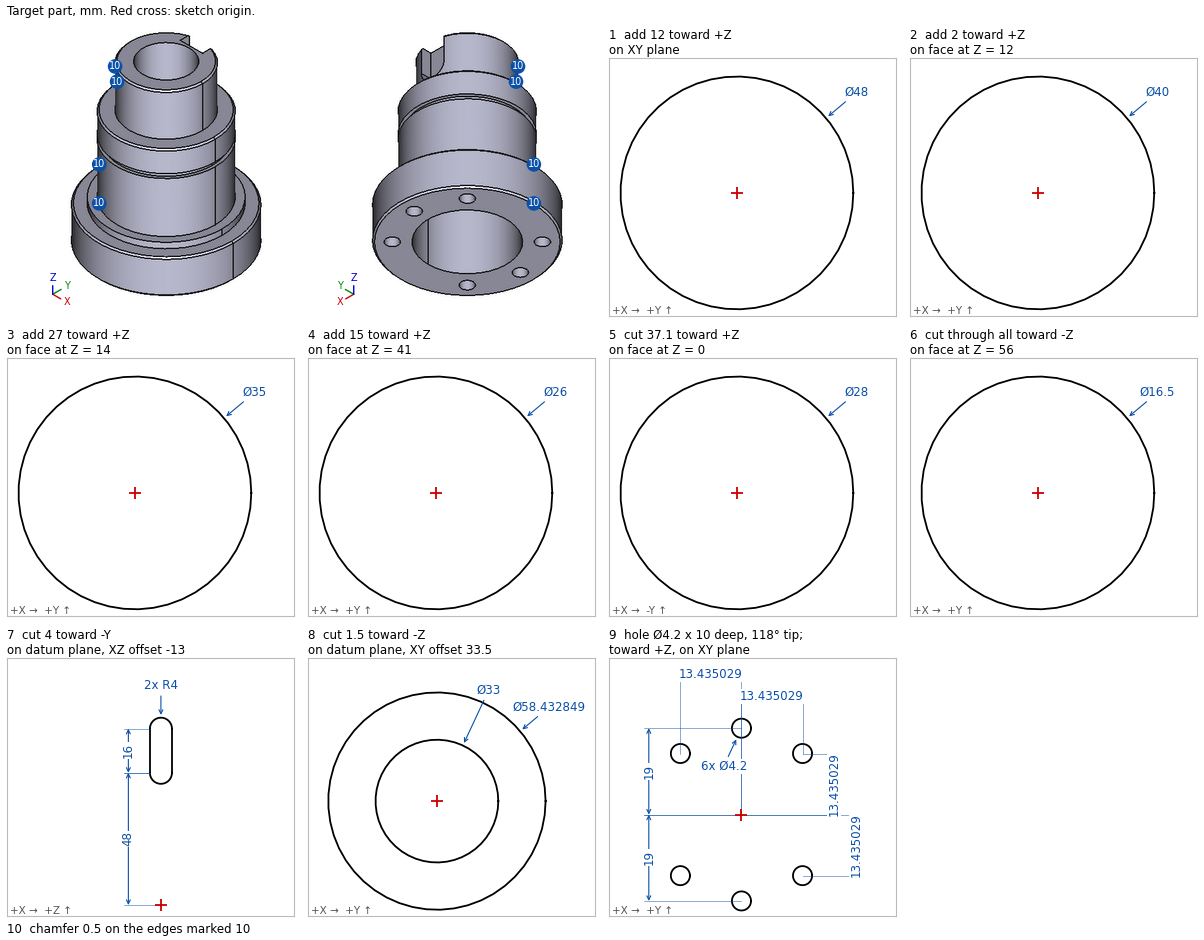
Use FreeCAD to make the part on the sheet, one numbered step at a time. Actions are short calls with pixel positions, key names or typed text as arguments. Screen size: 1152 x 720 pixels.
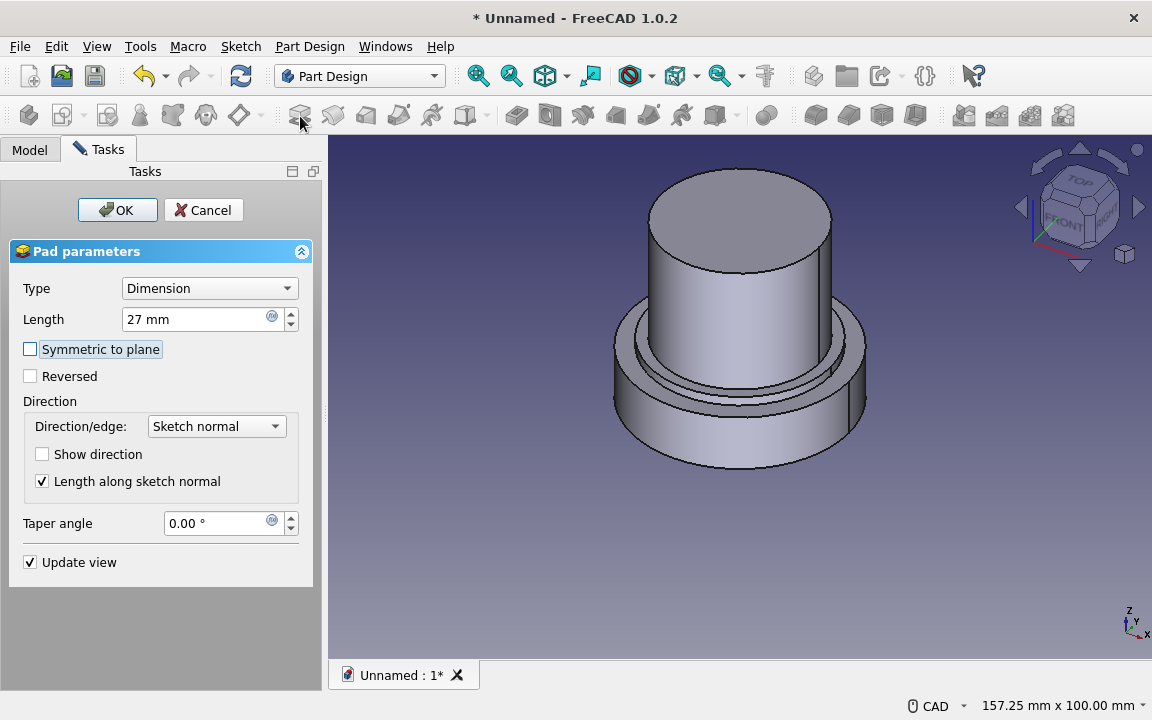
click(118, 210)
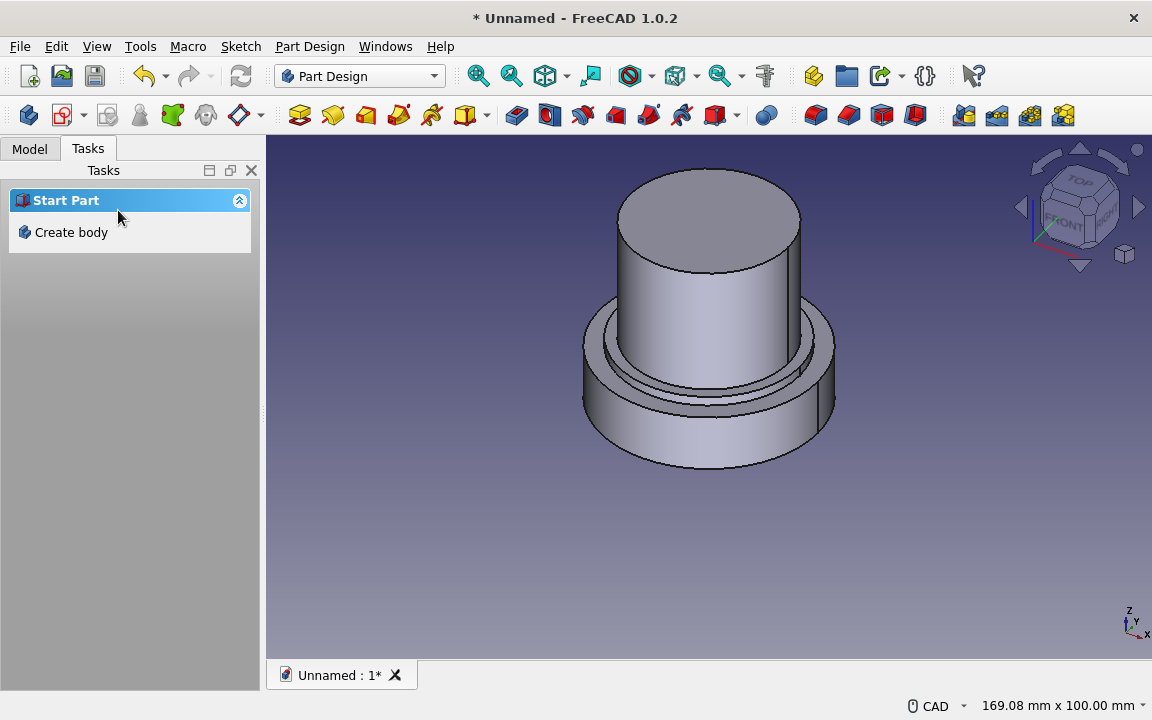
click(479, 76)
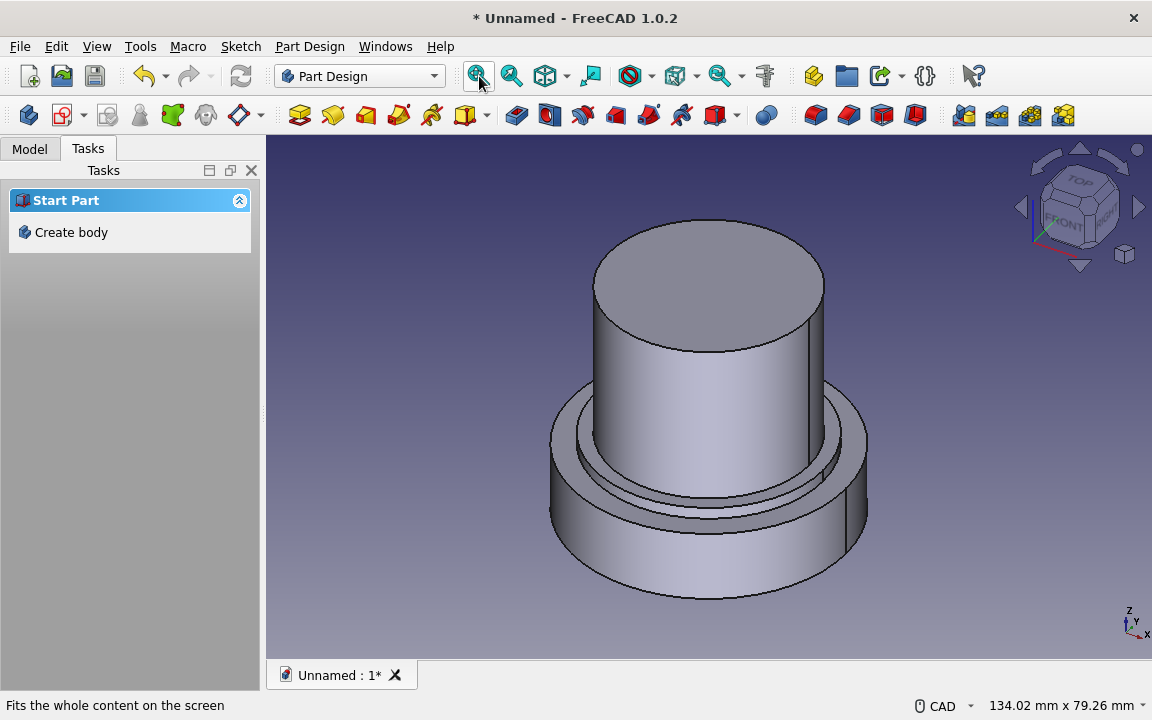
click(709, 285)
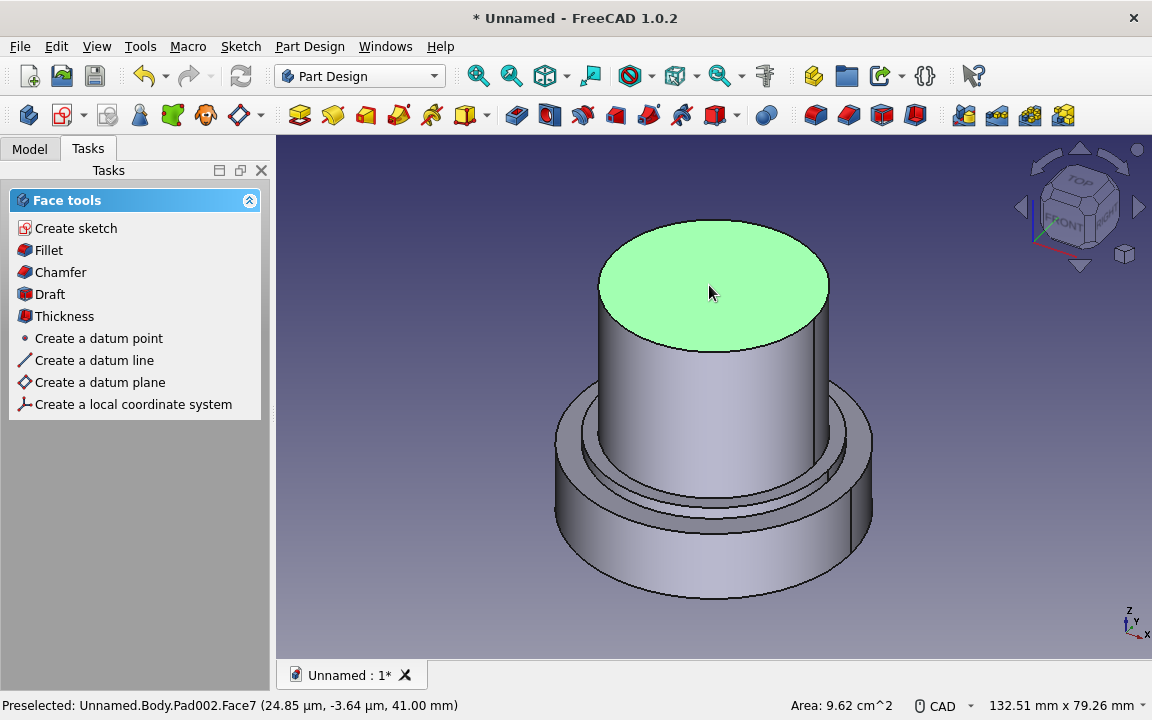
click(62, 116)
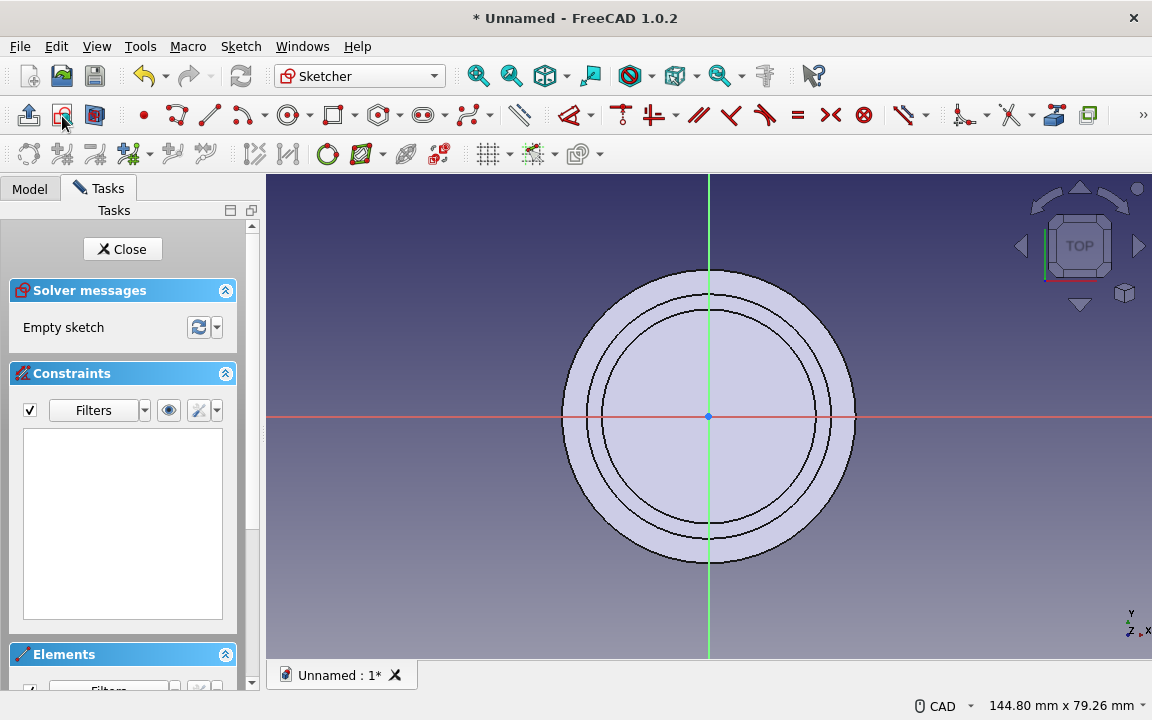
scroll(792, 416, up, 3)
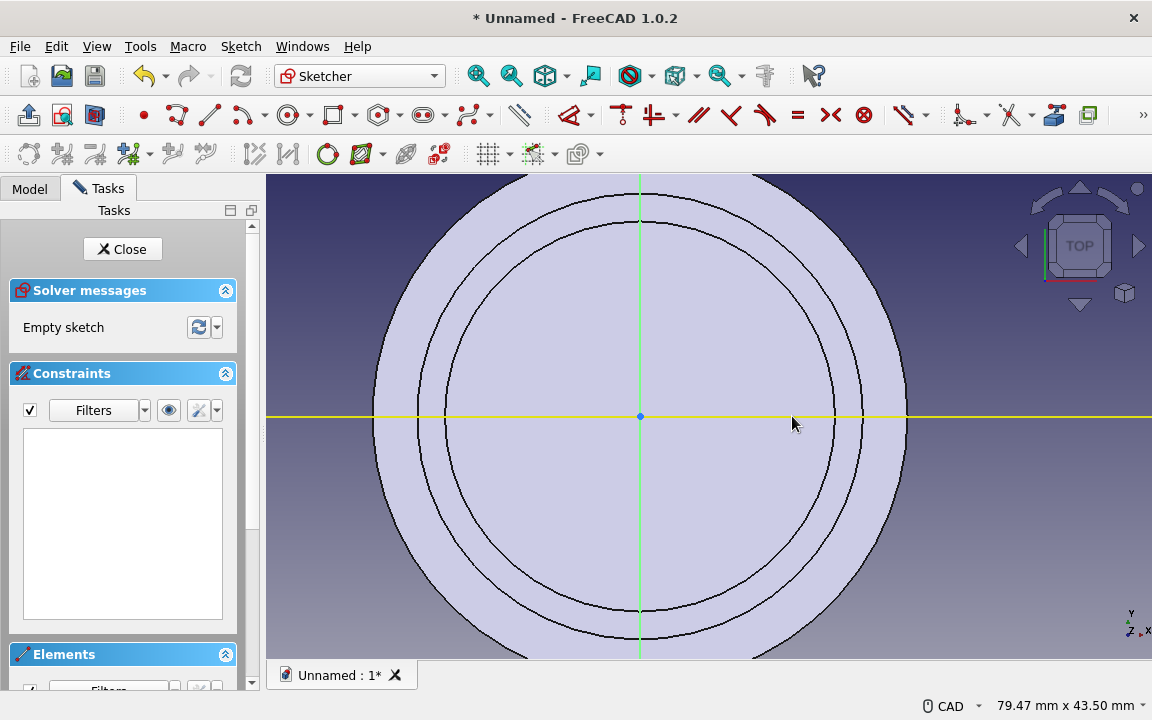
key(g)
key(c)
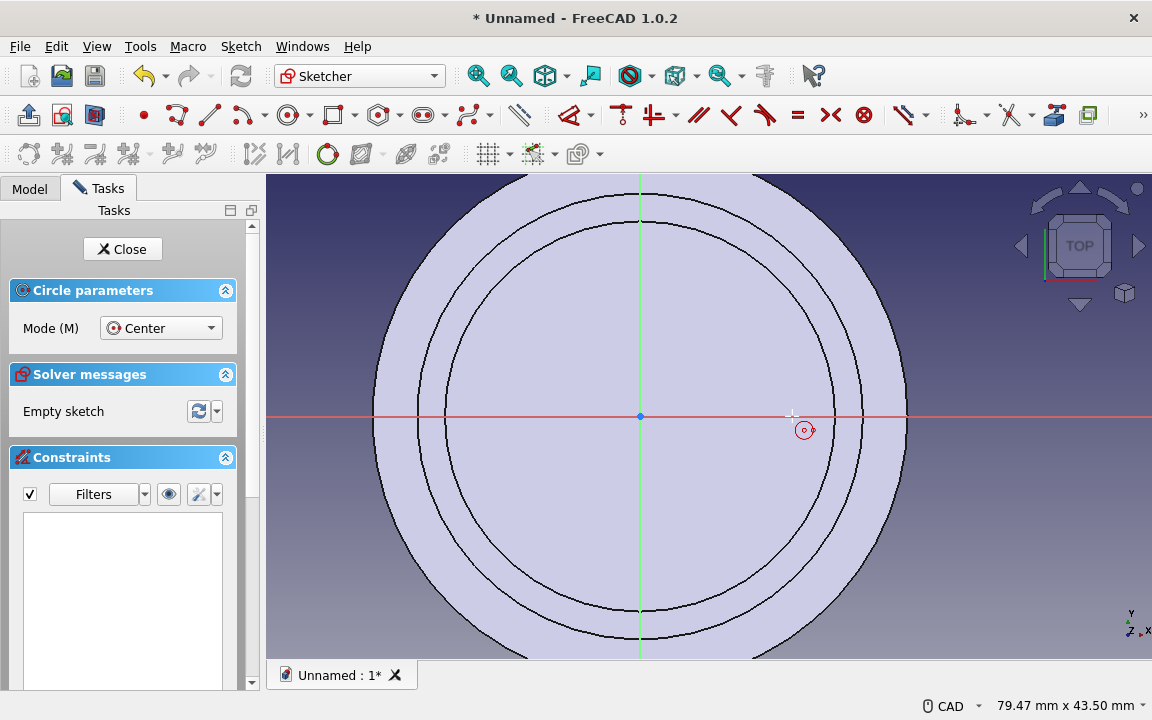
click(640, 416)
click(743, 314)
key(Escape)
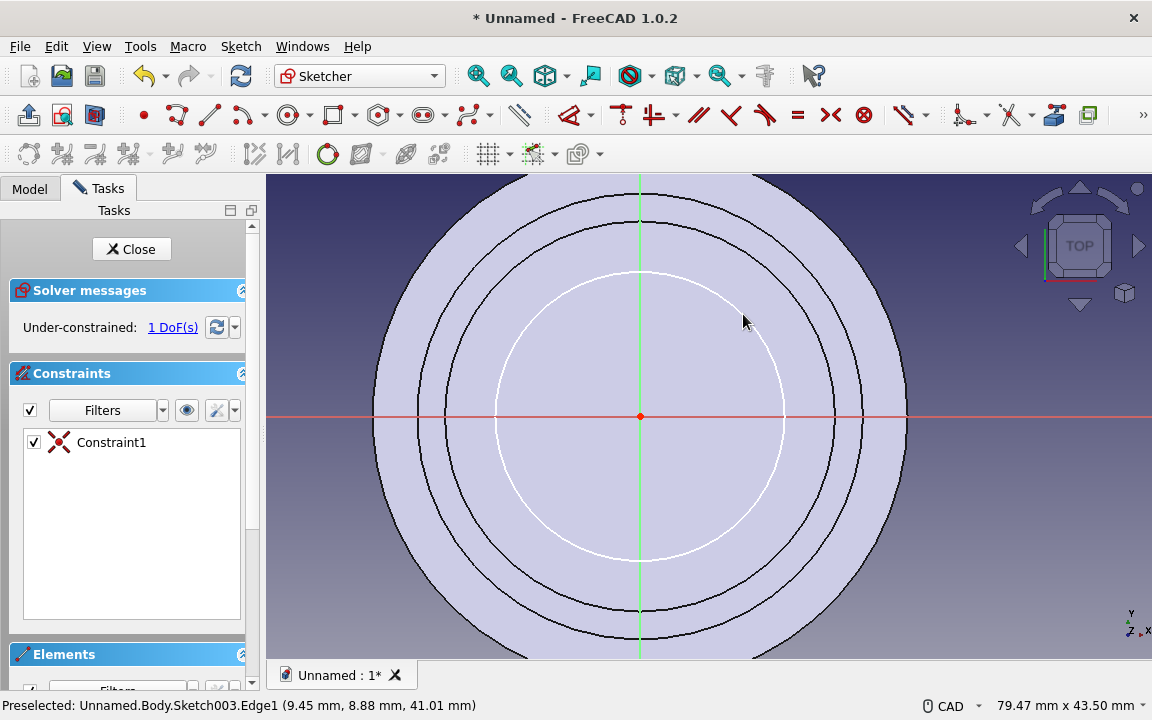
click(742, 314)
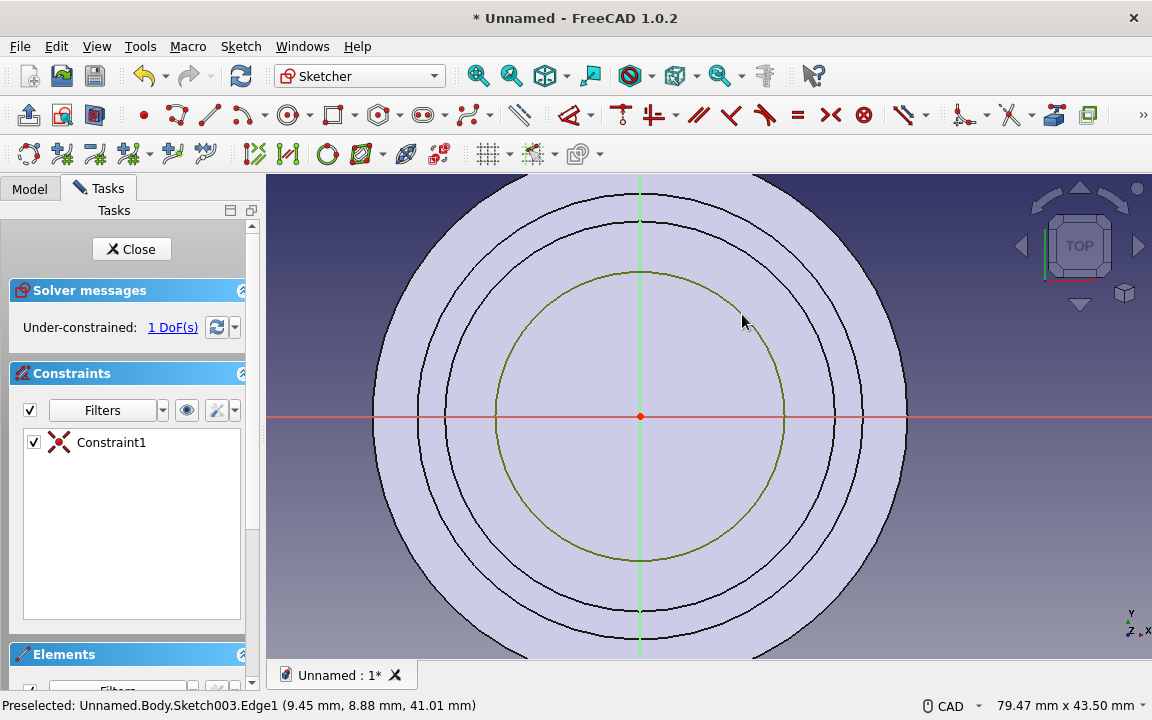
key(k)
key(o)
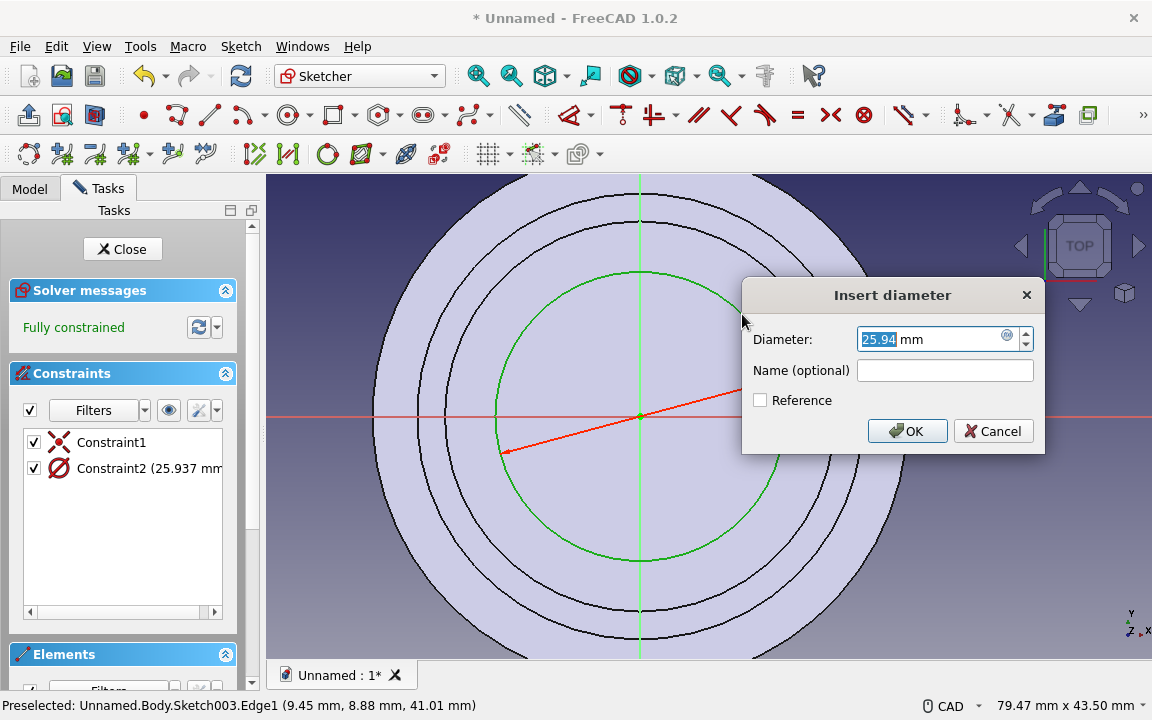
text(26)
key(Return)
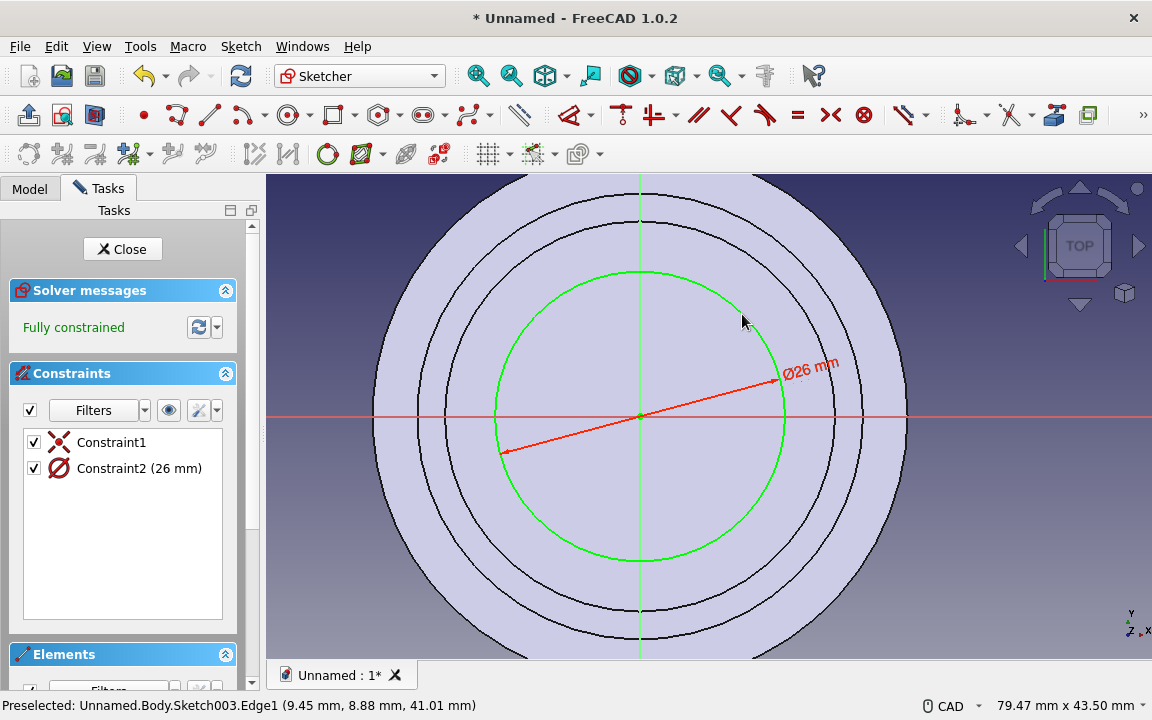
click(123, 249)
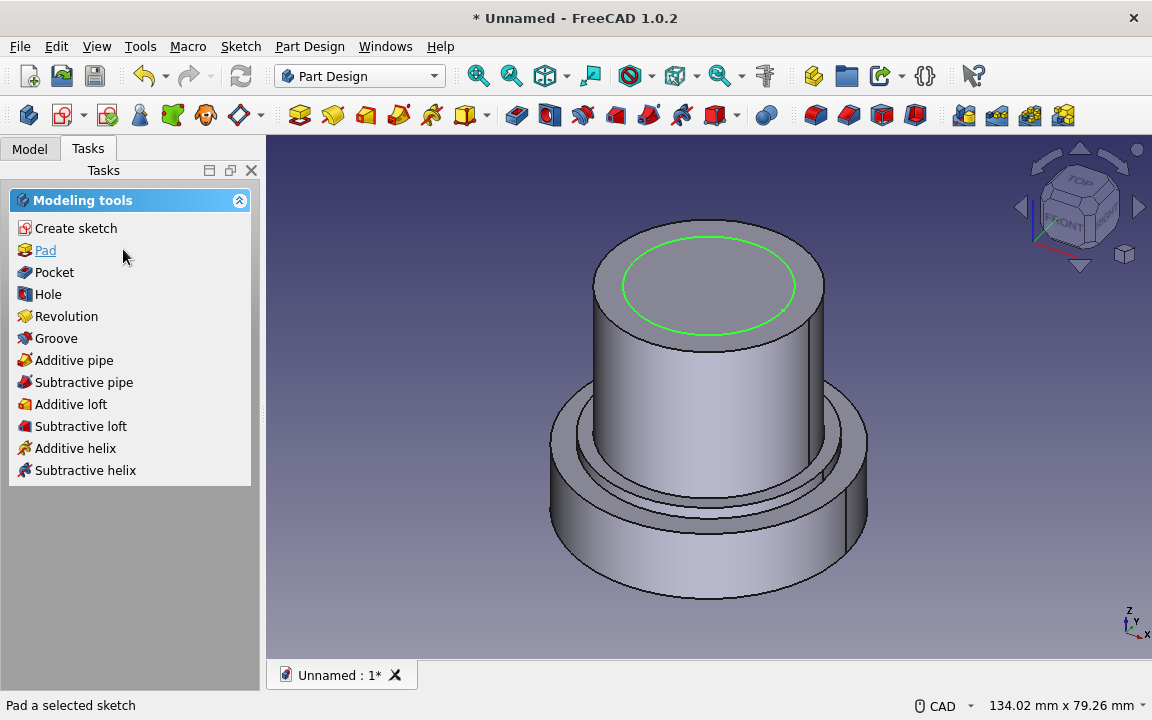
click(300, 116)